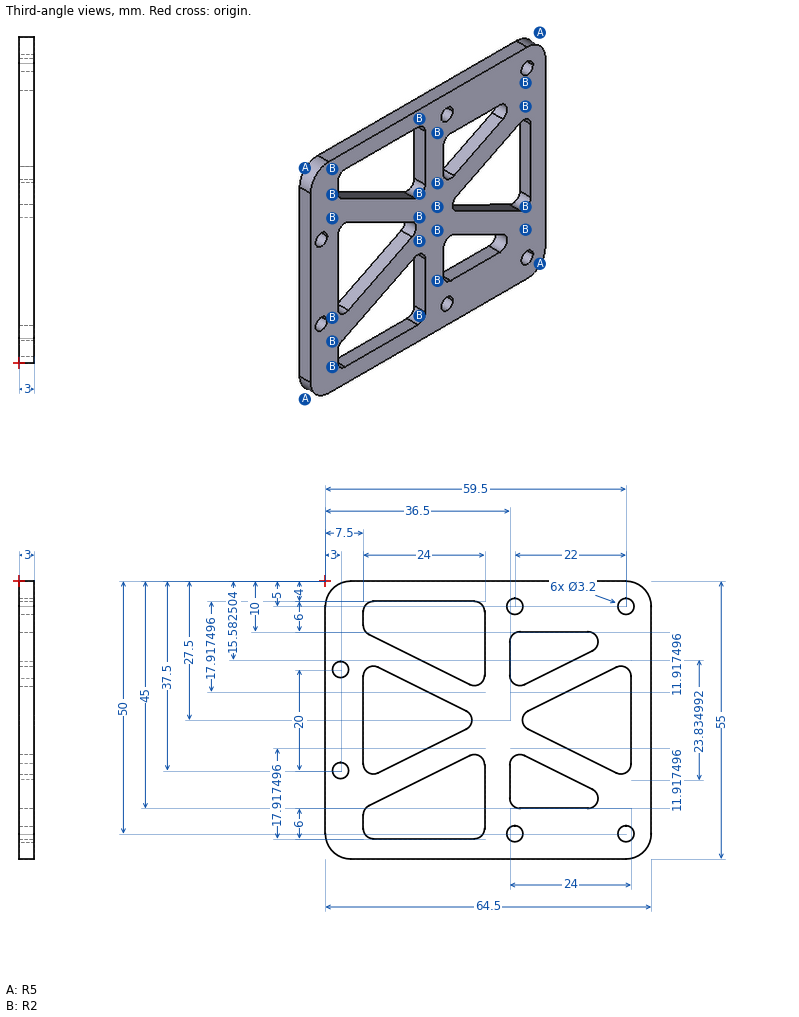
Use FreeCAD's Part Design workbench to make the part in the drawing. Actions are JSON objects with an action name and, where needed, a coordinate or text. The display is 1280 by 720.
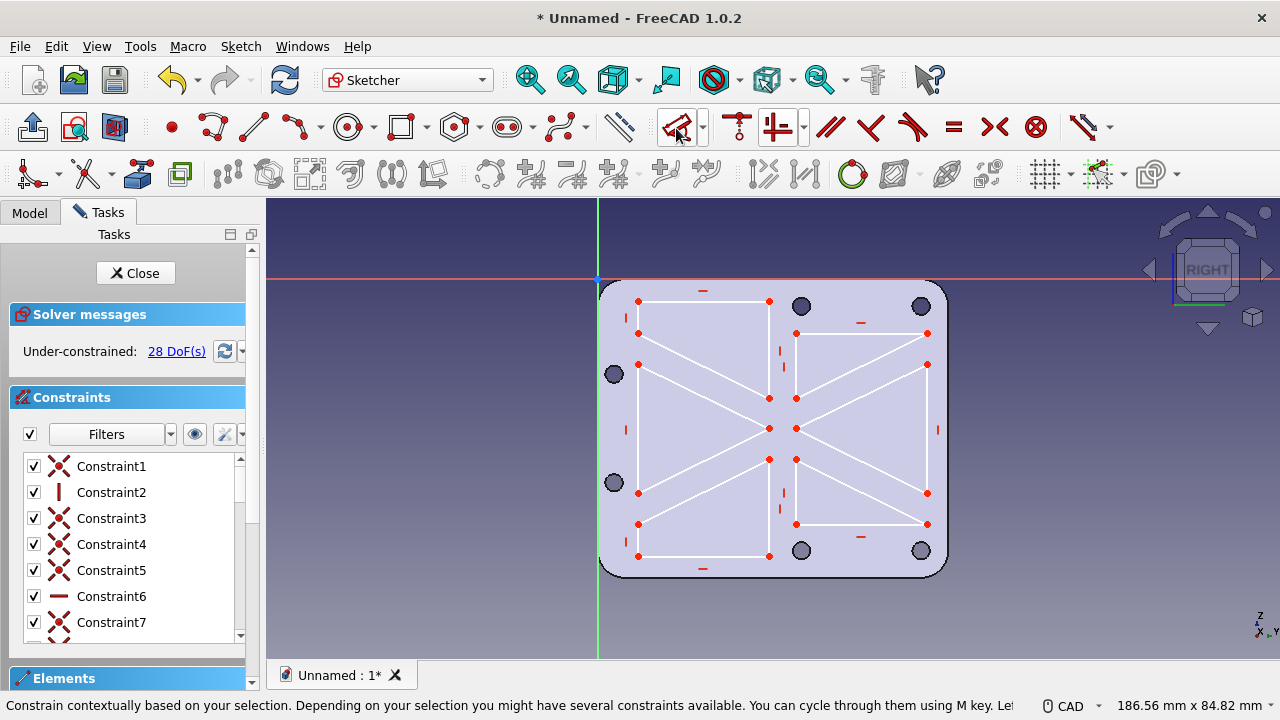
{"action": "scroll", "coordinate": [638, 324], "scroll_direction": "up", "scroll_amount": 2}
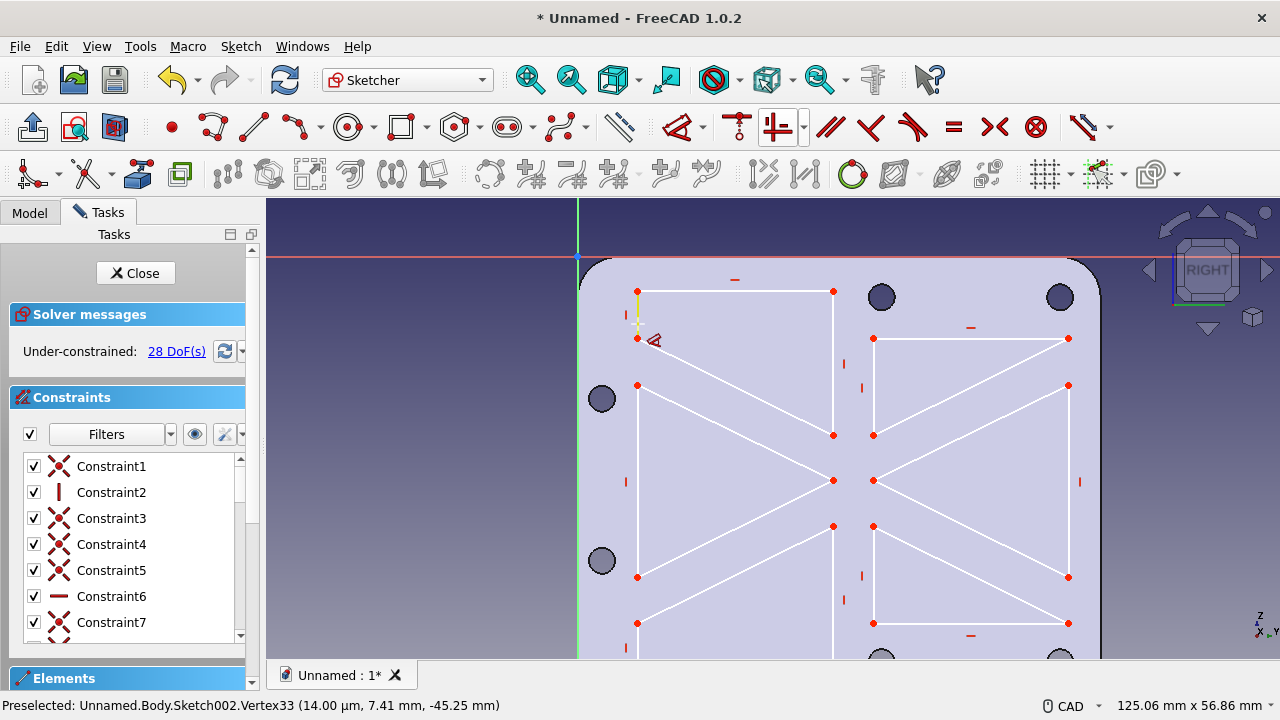
{"action": "left_click", "coordinate": [638, 324]}
{"action": "left_click", "coordinate": [604, 315]}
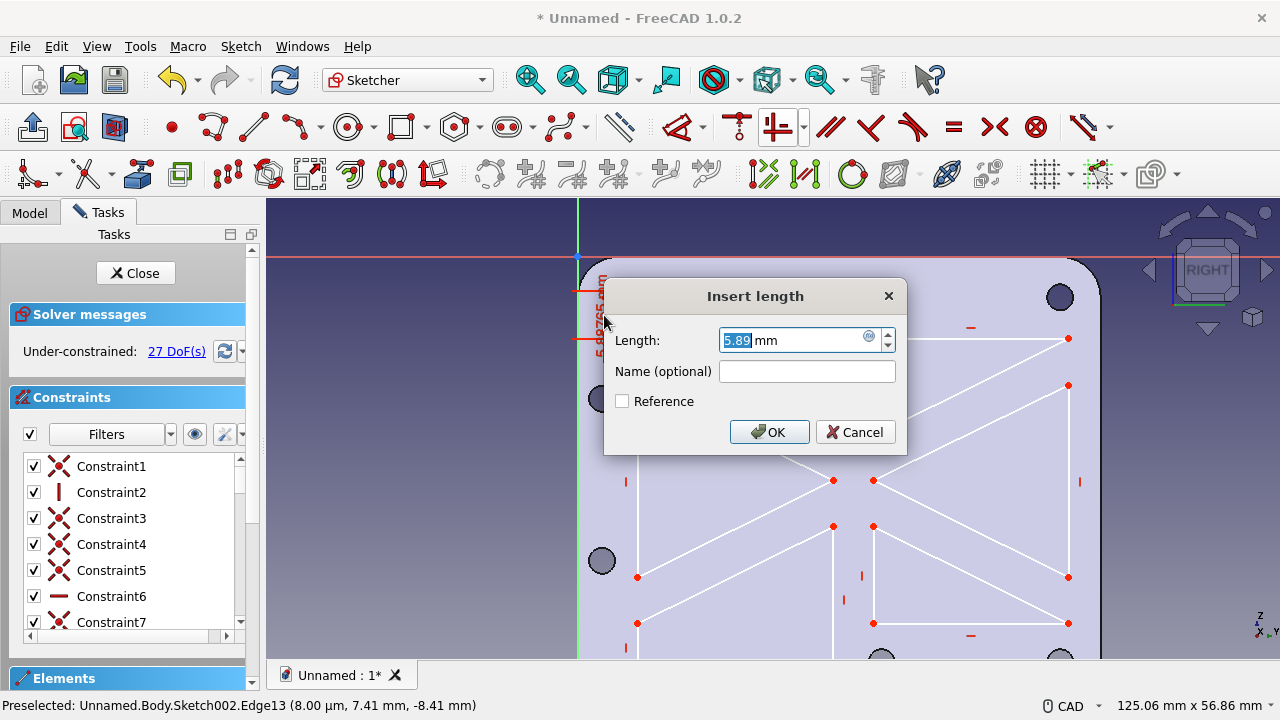
{"action": "type", "text": "6"}
{"action": "key", "text": "Return"}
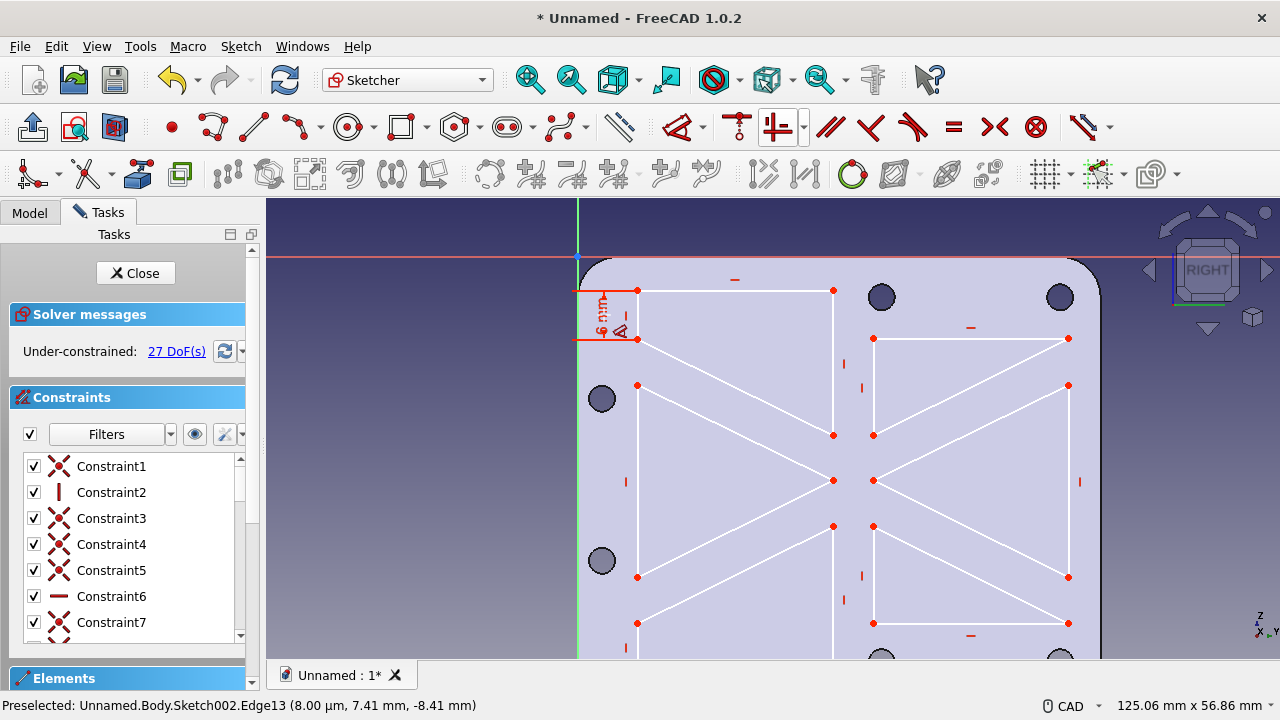
{"action": "scroll", "coordinate": [464, 357], "scroll_direction": "down", "scroll_amount": 2}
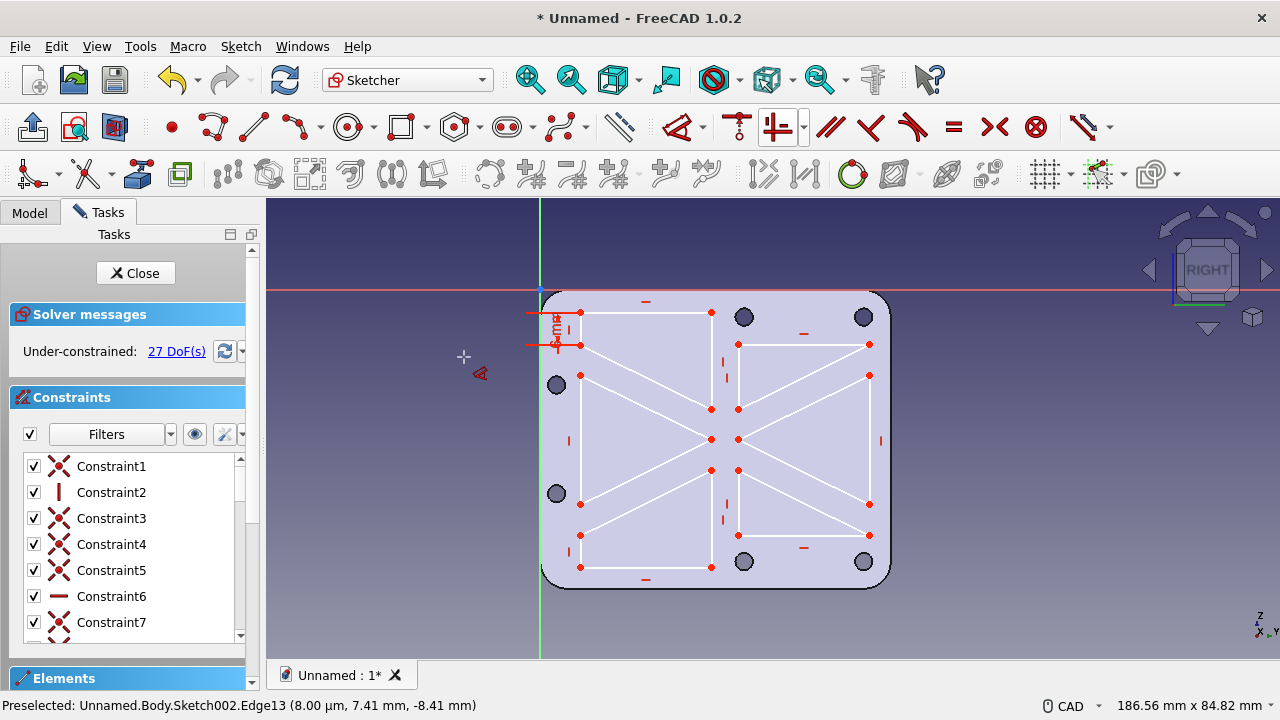
{"action": "scroll", "coordinate": [581, 558], "scroll_direction": "up", "scroll_amount": 2}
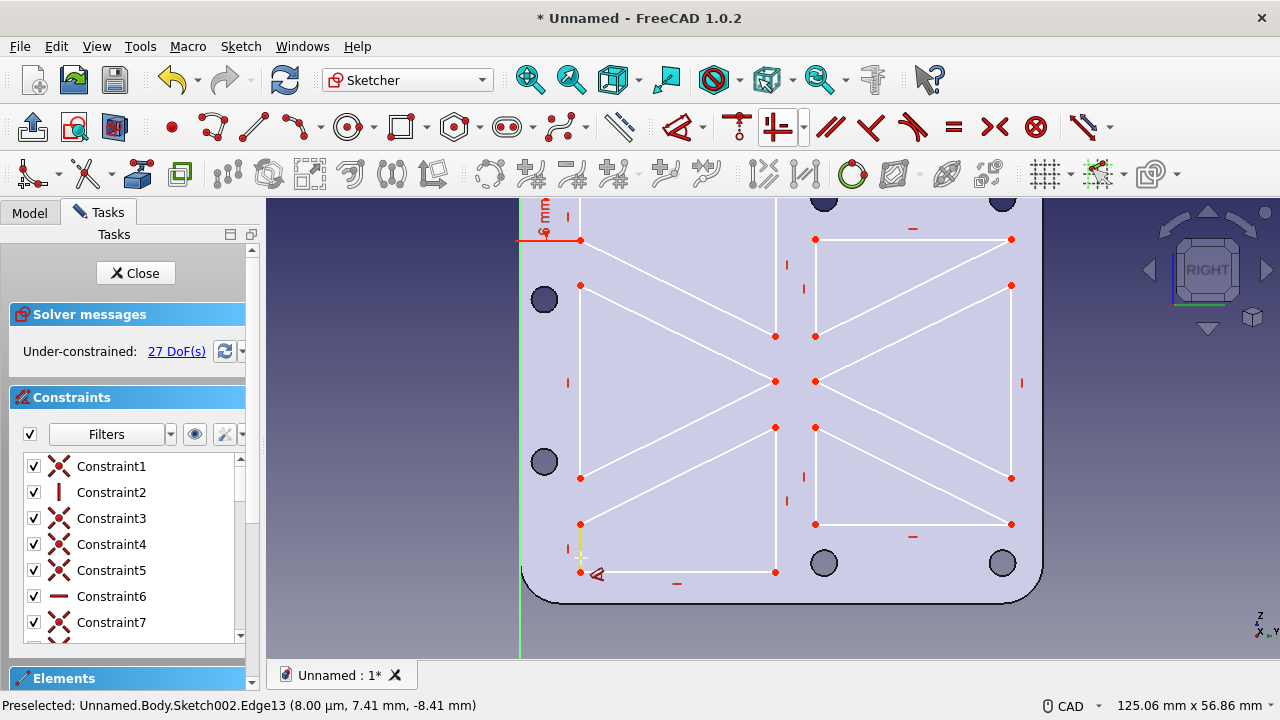
{"action": "left_click", "coordinate": [580, 558]}
{"action": "left_click", "coordinate": [546, 549]}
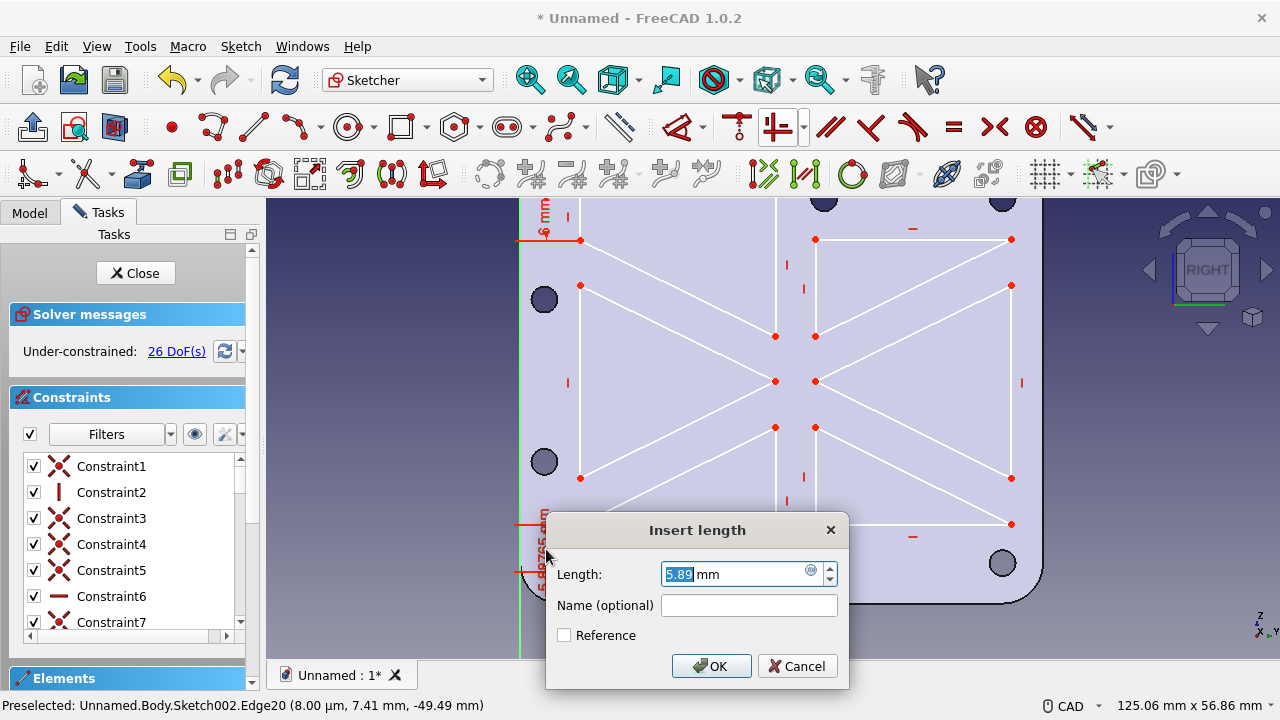
{"action": "type", "text": "6"}
{"action": "key", "text": "Return"}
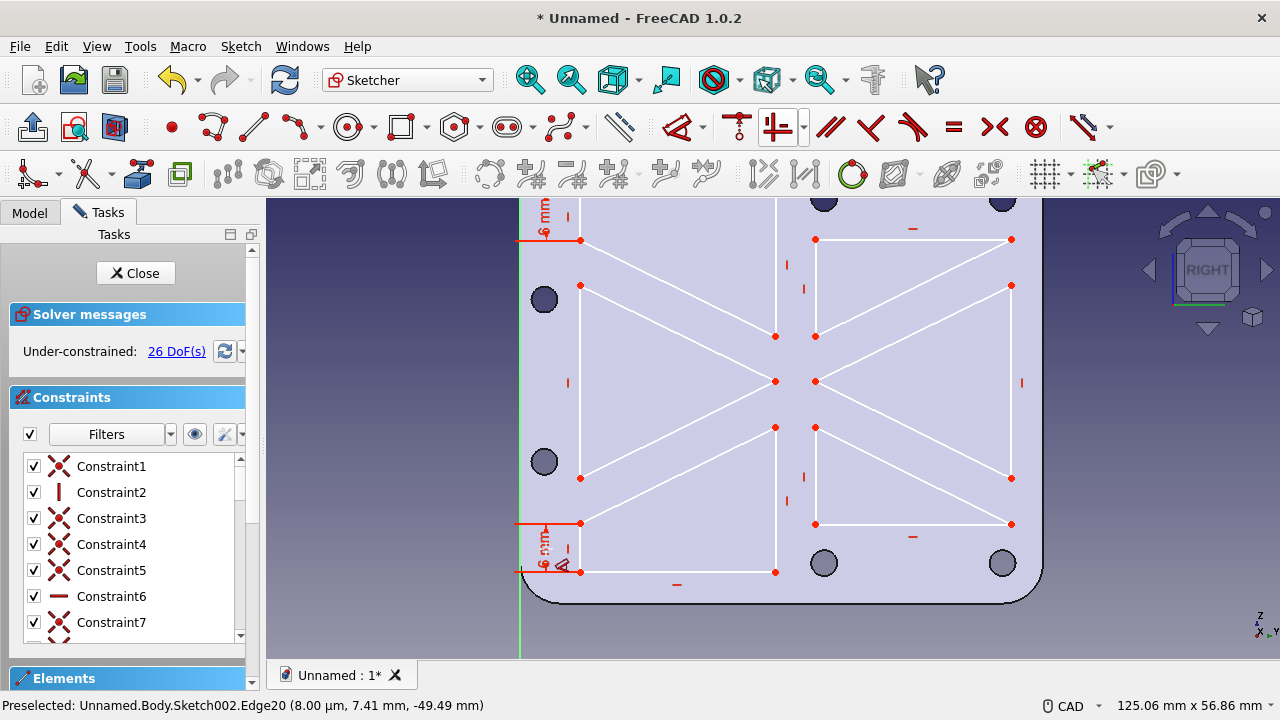
{"action": "left_click", "coordinate": [953, 525]}
{"action": "left_click", "coordinate": [914, 559]}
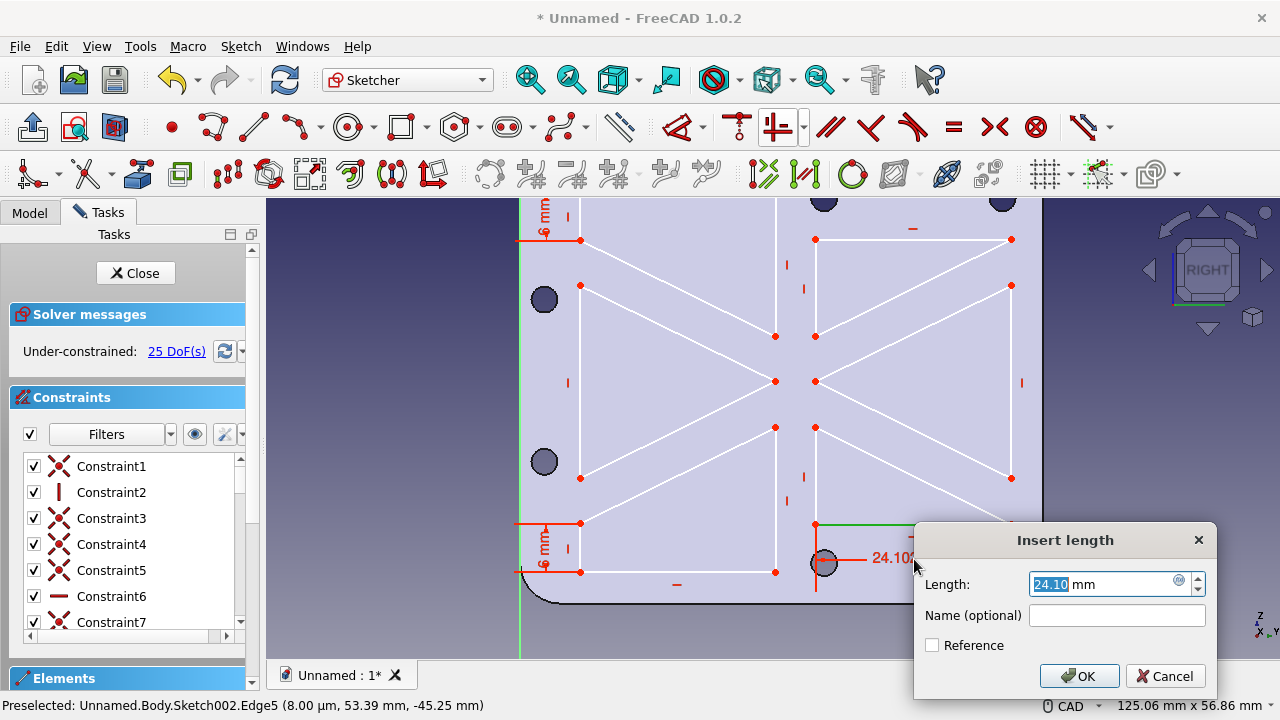
{"action": "type", "text": "24"}
{"action": "key", "text": "Return"}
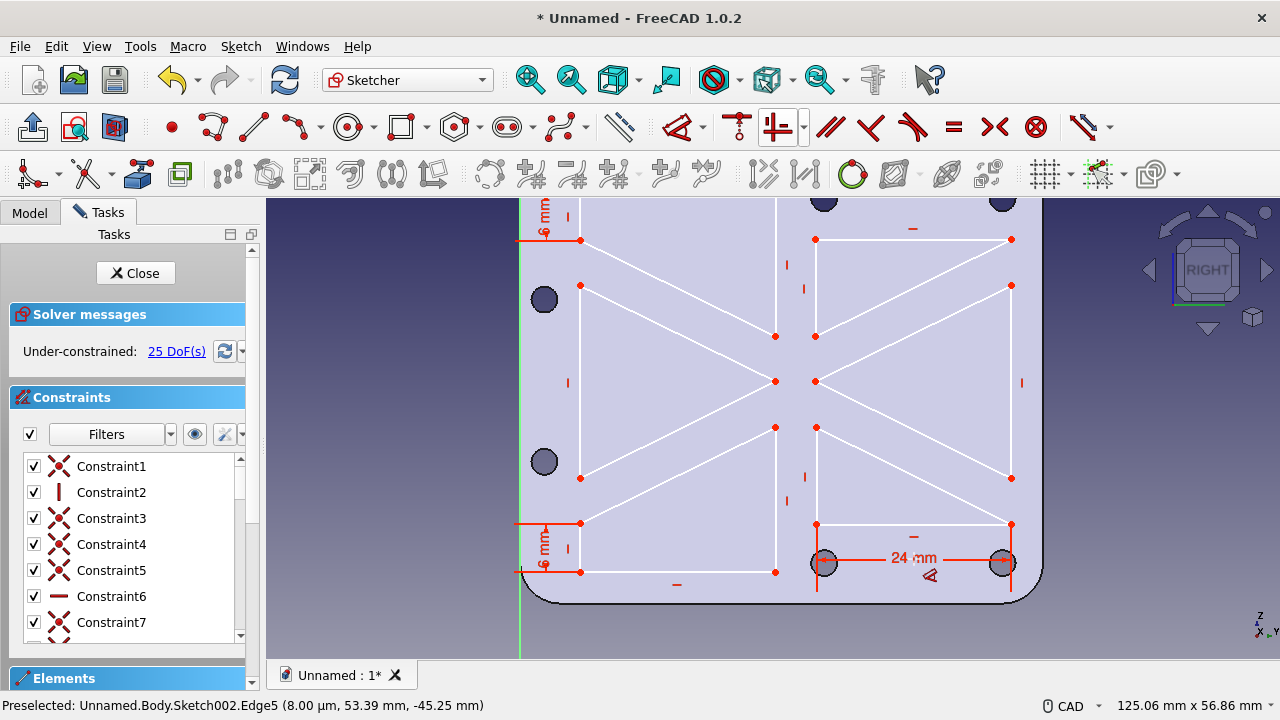
{"action": "left_click", "coordinate": [875, 240]}
{"action": "left_click", "coordinate": [869, 274]}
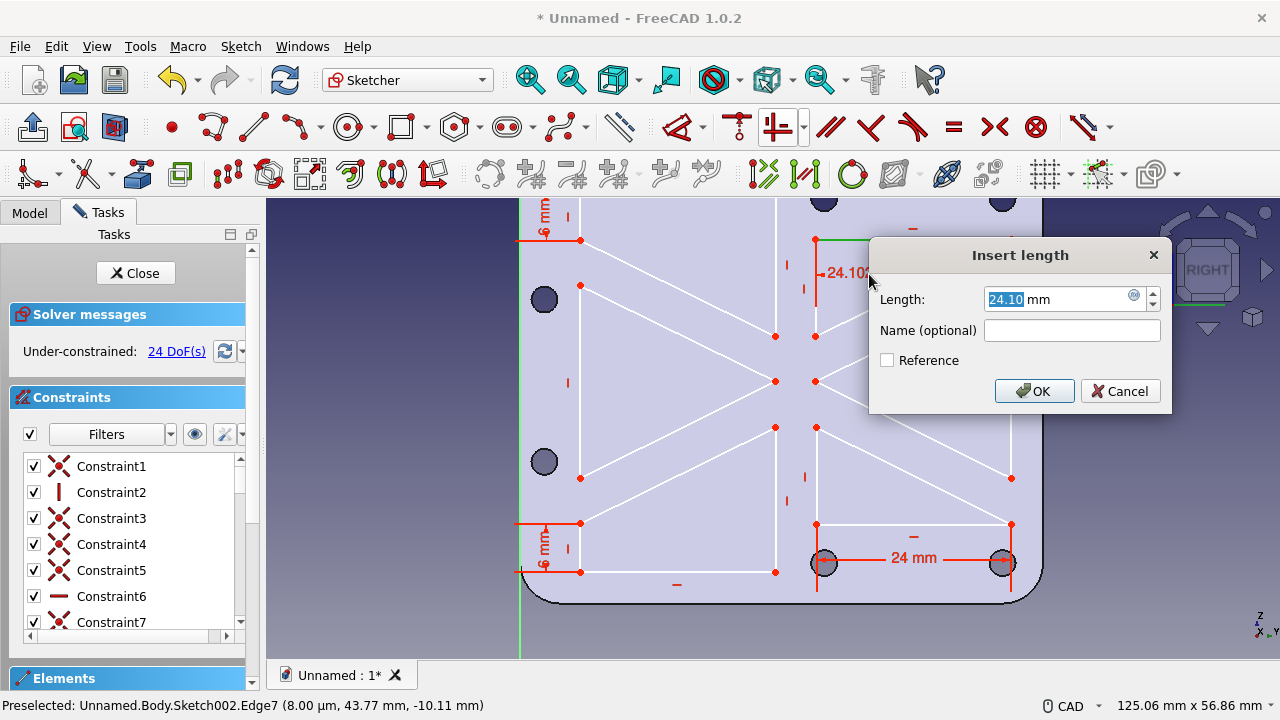
{"action": "type", "text": "24"}
{"action": "key", "text": "Return"}